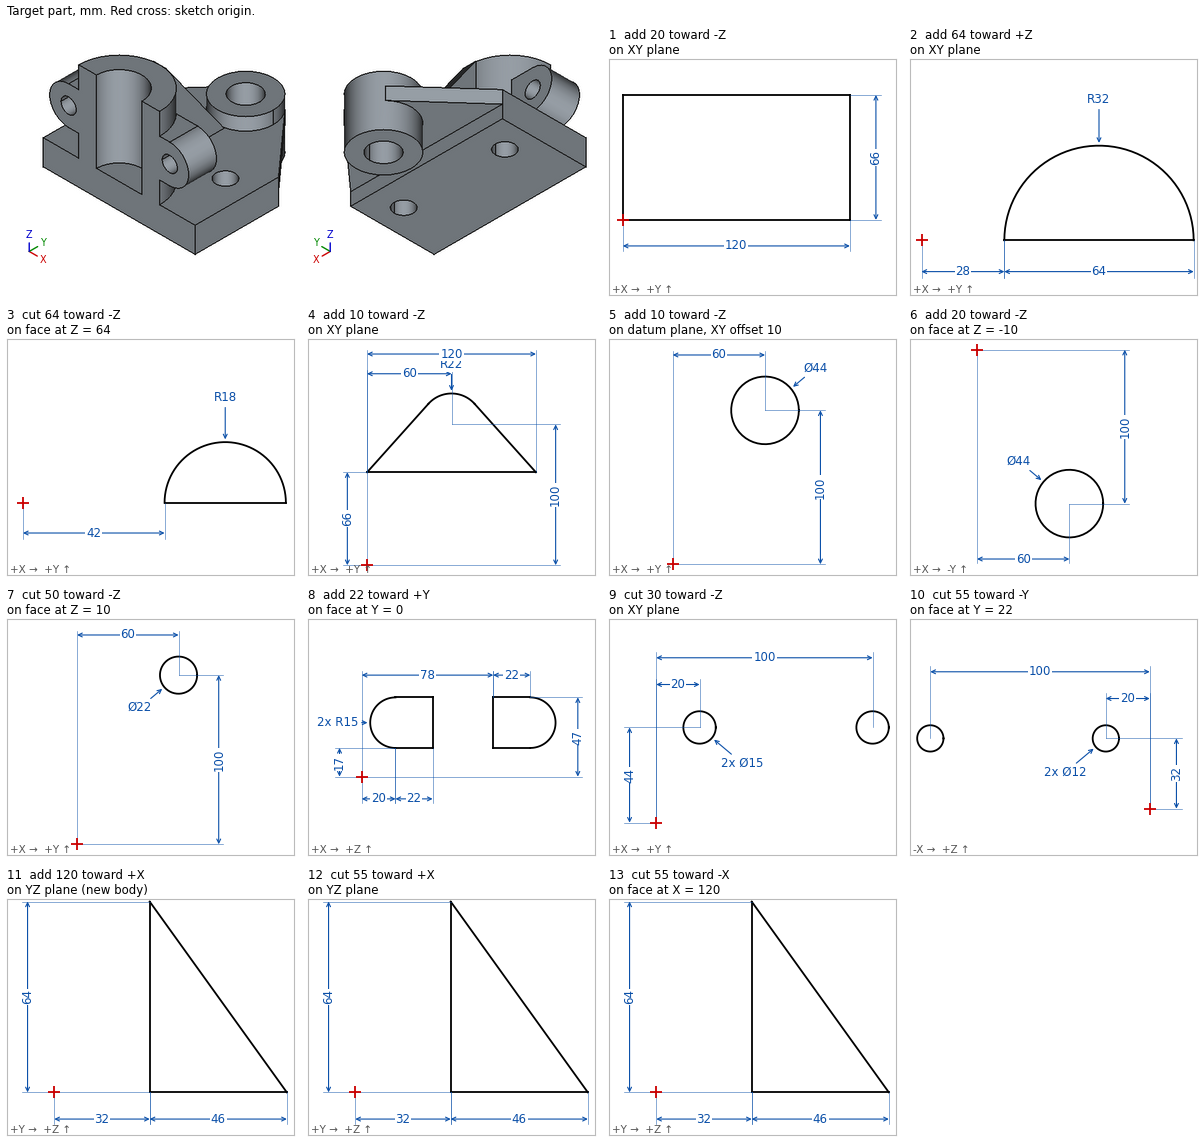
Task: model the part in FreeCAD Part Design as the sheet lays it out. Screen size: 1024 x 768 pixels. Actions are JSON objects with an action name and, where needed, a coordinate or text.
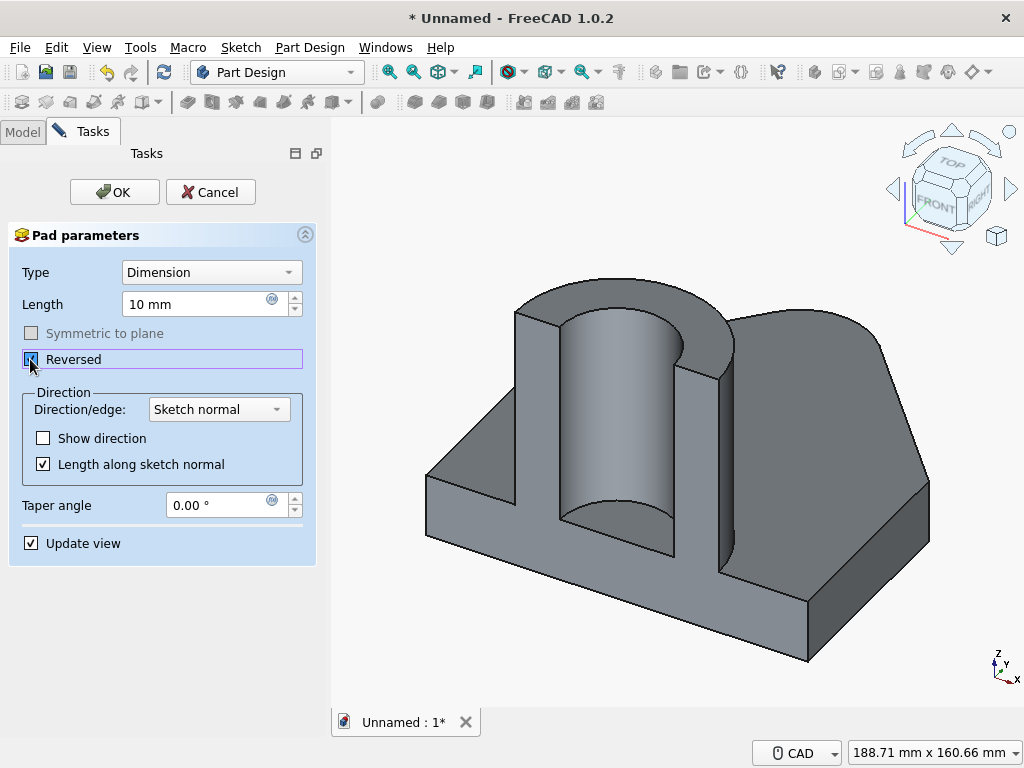
{"action": "left_click", "coordinate": [115, 192]}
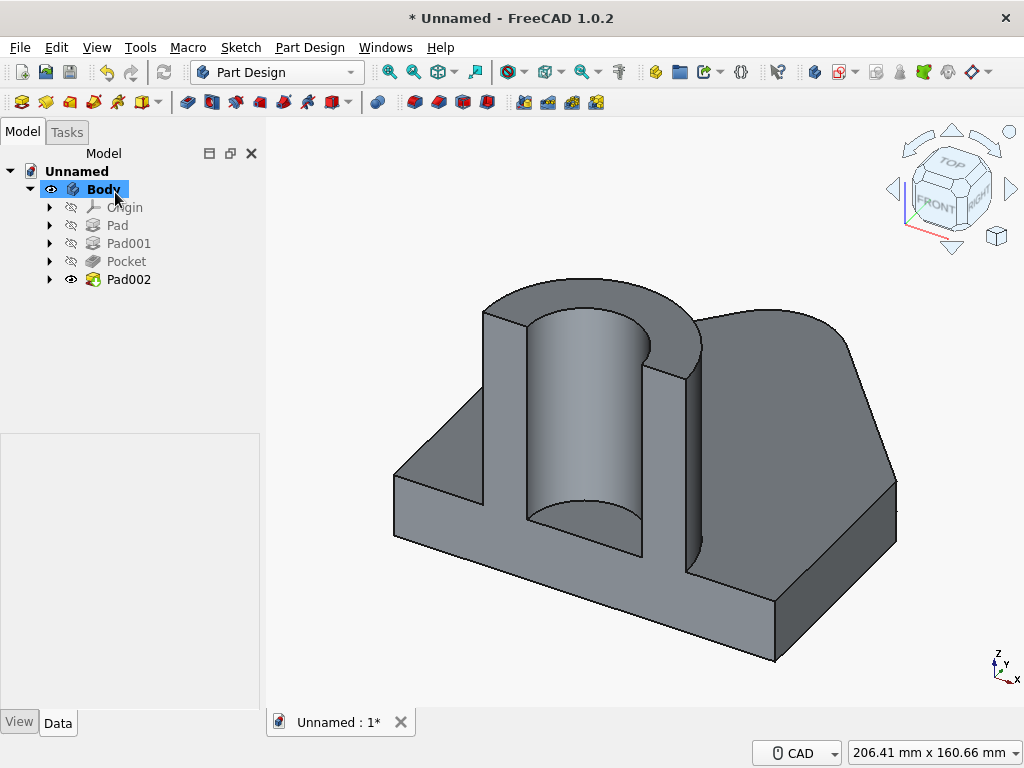
{"action": "left_click", "coordinate": [390, 72]}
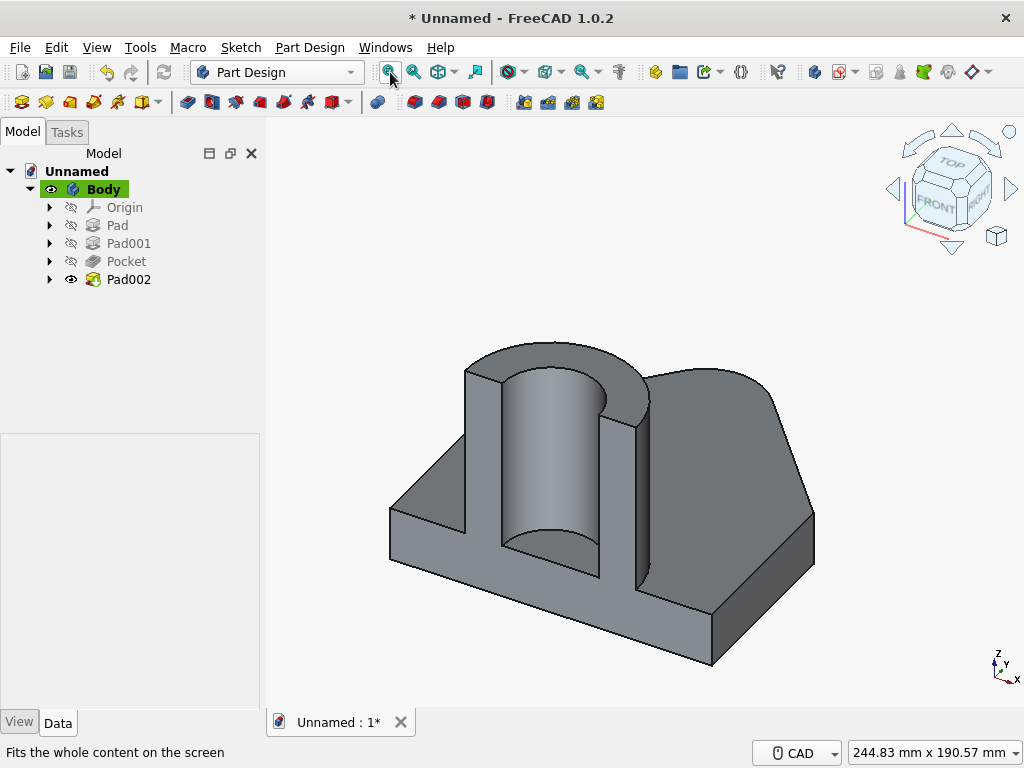
{"action": "left_click", "coordinate": [50, 207]}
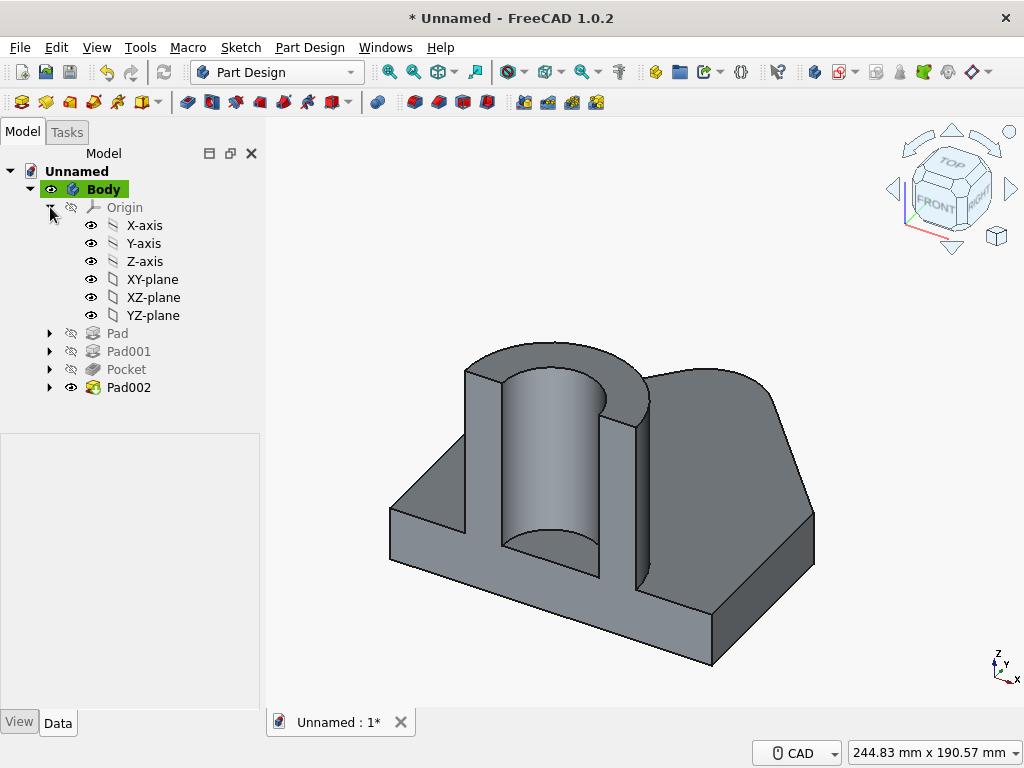
{"action": "left_click", "coordinate": [136, 279]}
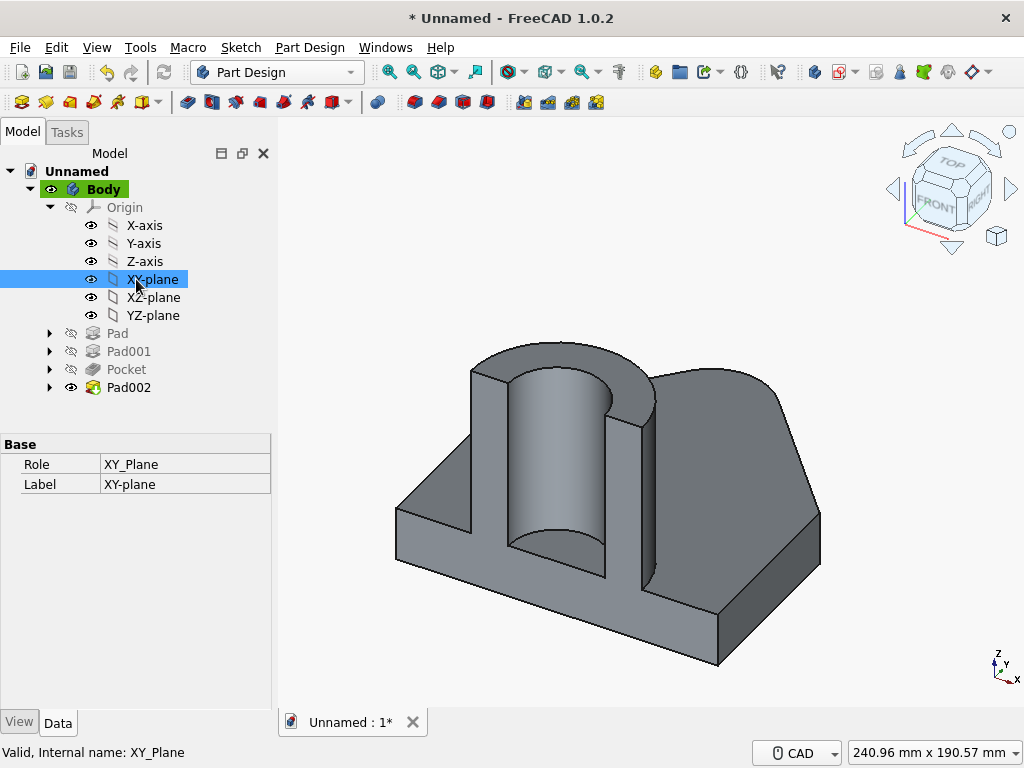
{"action": "left_click", "coordinate": [972, 72]}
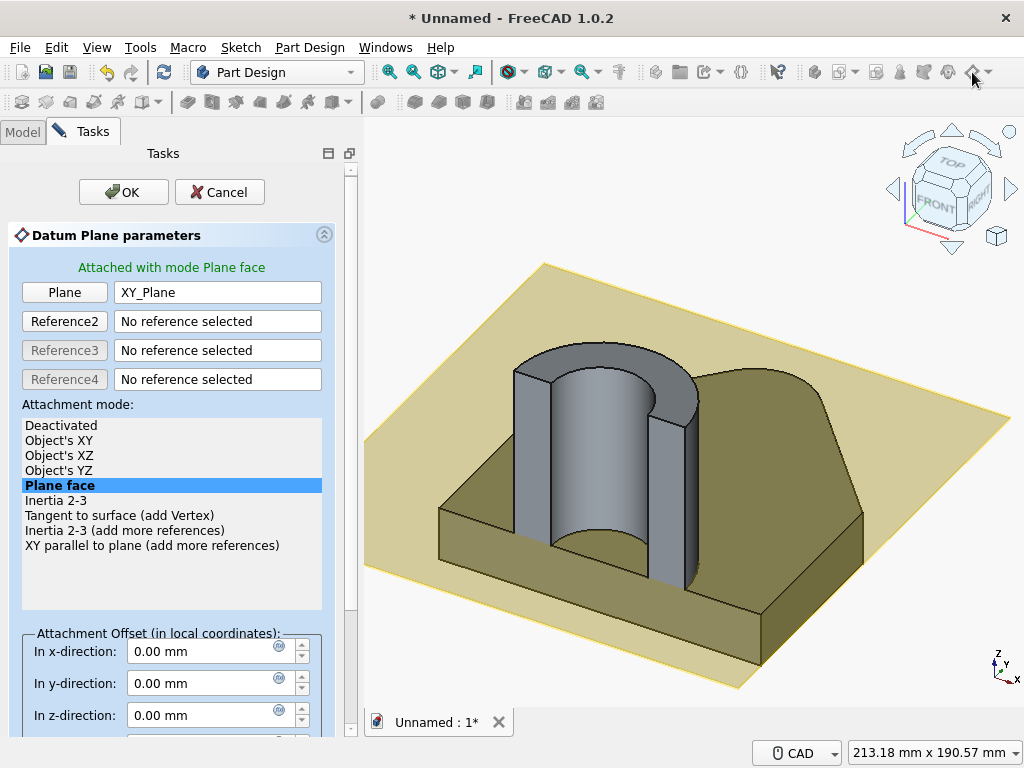
{"action": "triple_click", "coordinate": [210, 715]}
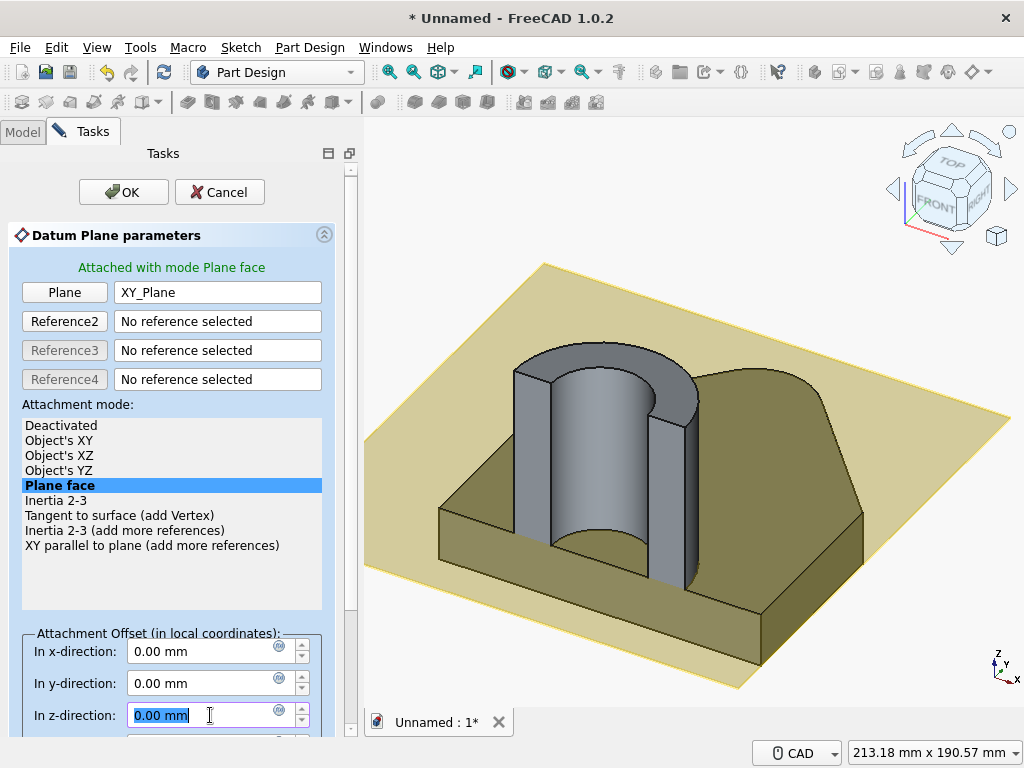
{"action": "type", "text": "10"}
{"action": "key", "text": "Tab"}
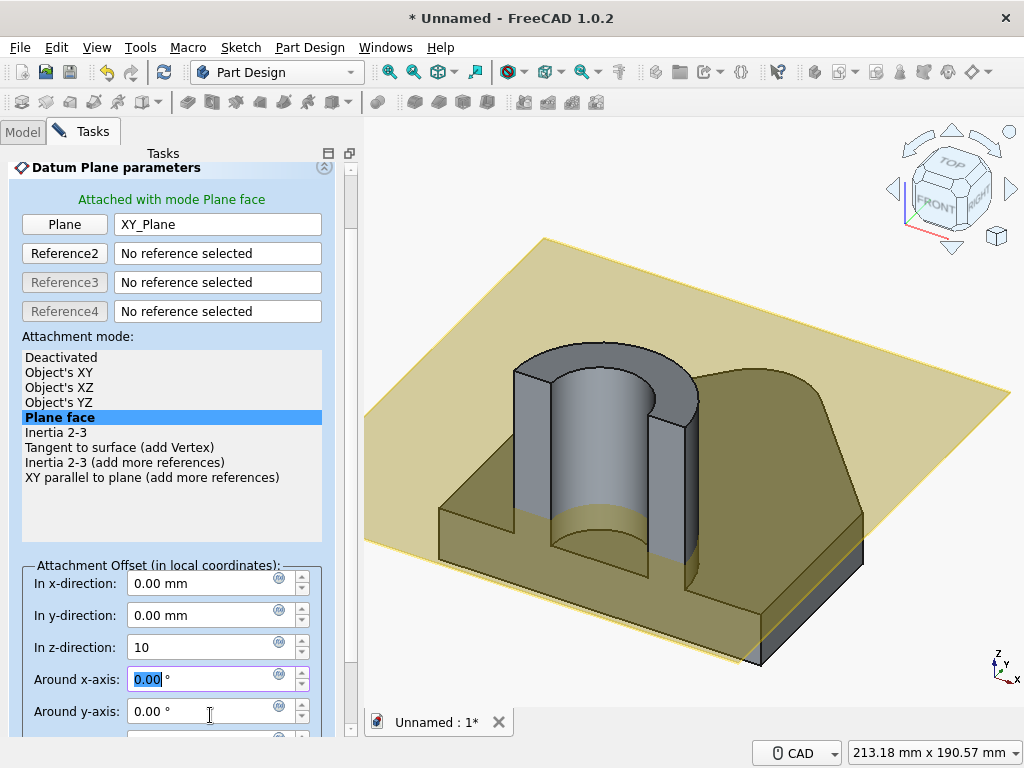
{"action": "scroll", "coordinate": [351, 450], "scroll_direction": "up", "scroll_amount": 2}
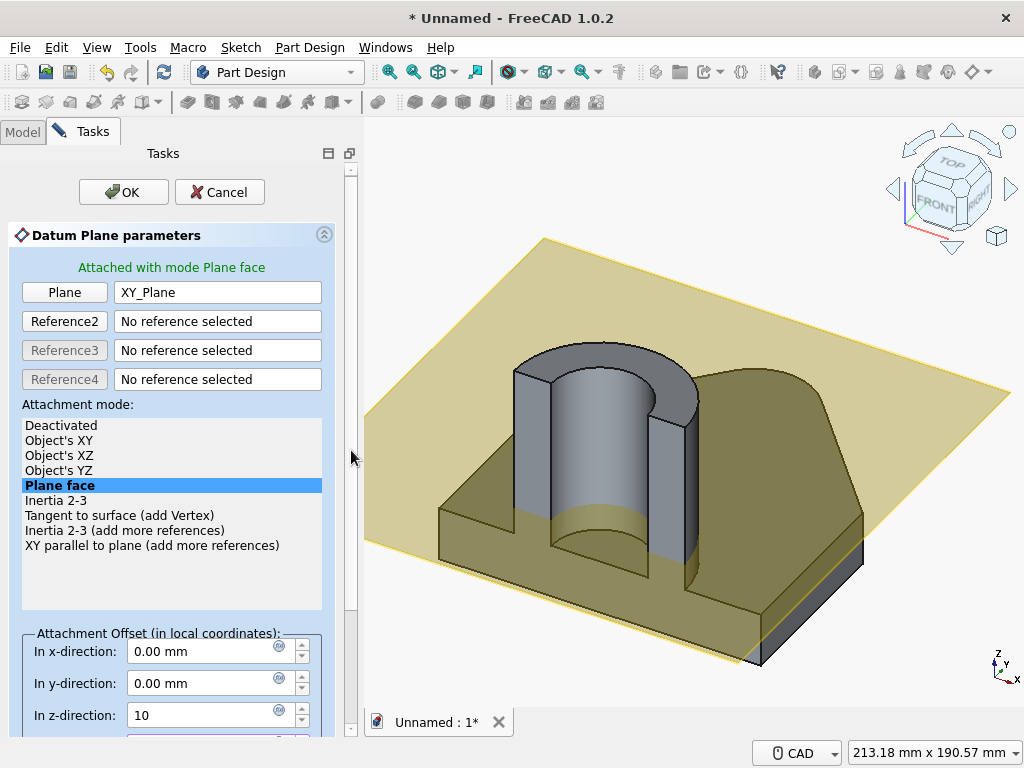
{"action": "left_click", "coordinate": [124, 192]}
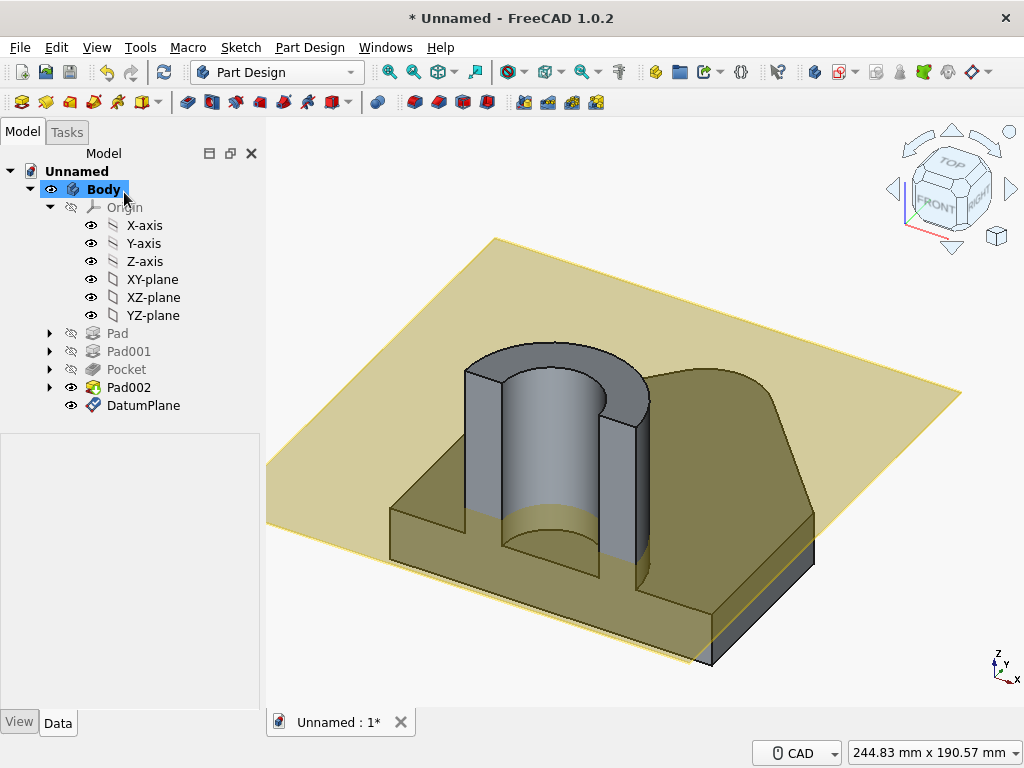
{"action": "left_click", "coordinate": [116, 405]}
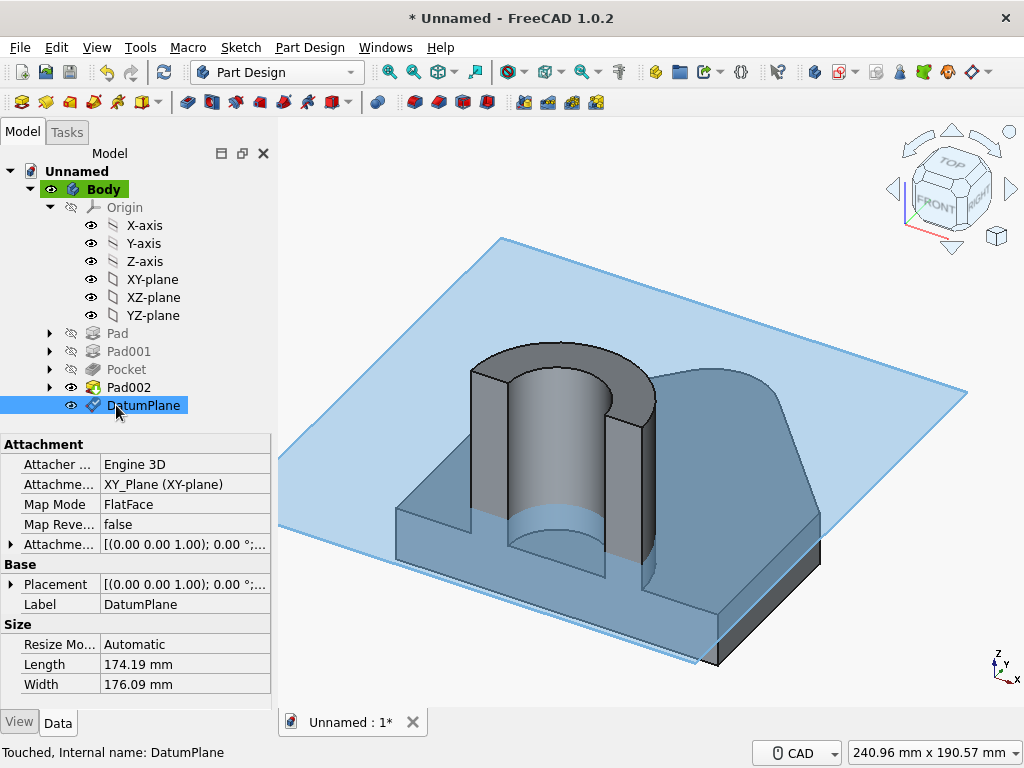
{"action": "left_click", "coordinate": [840, 72]}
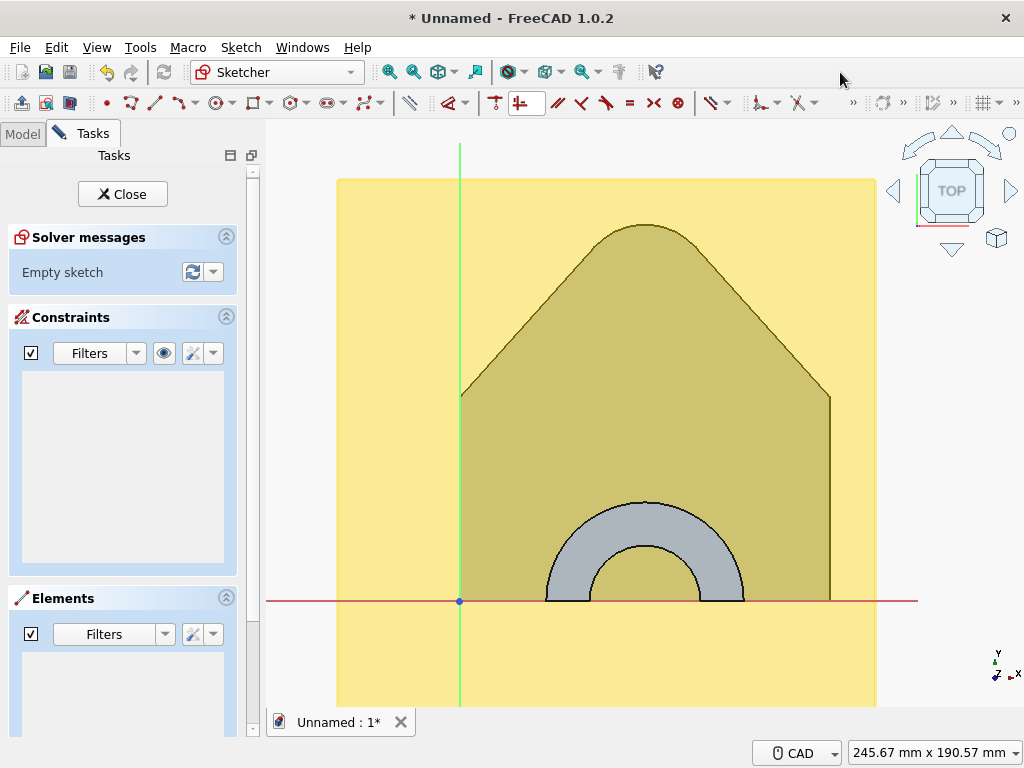
{"action": "left_click", "coordinate": [70, 104]}